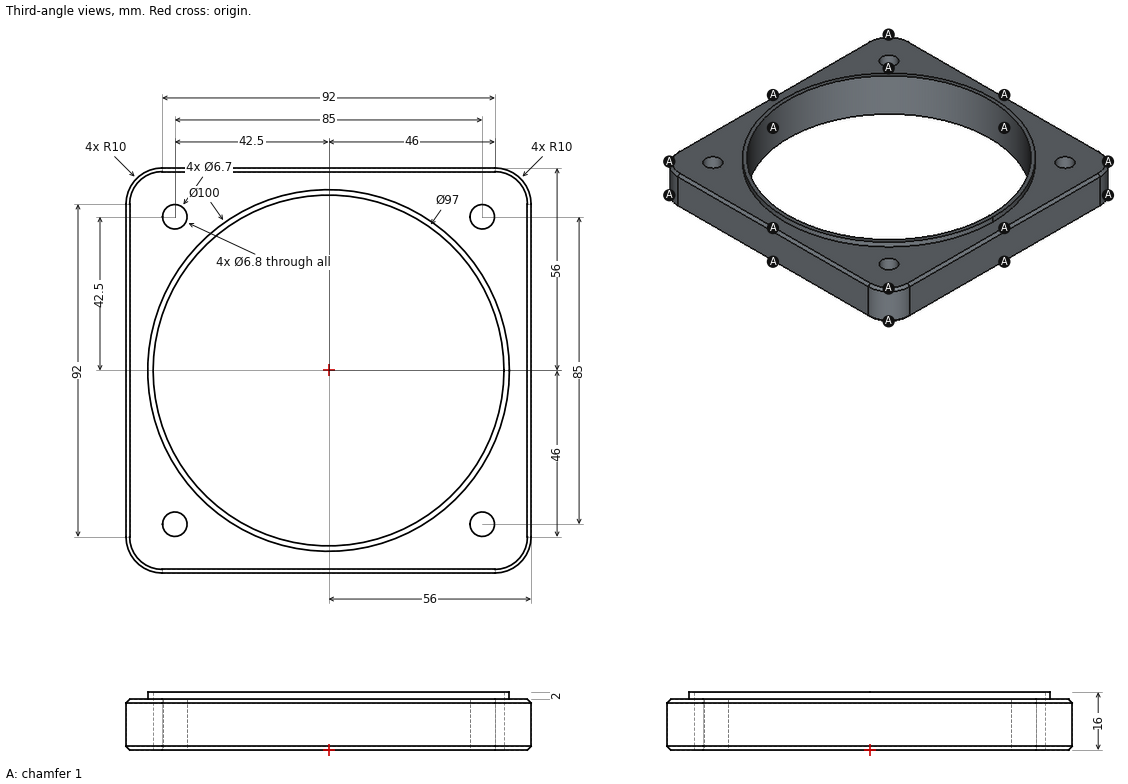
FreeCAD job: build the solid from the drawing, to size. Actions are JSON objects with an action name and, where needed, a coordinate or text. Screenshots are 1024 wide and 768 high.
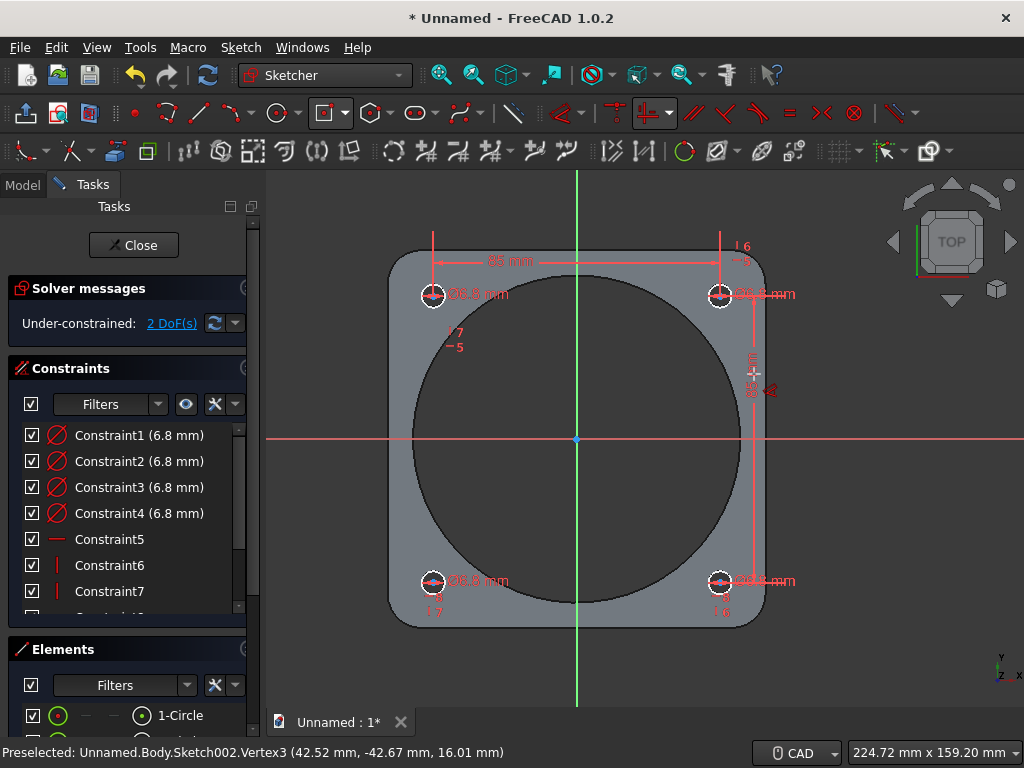
{"action": "left_click", "coordinate": [433, 296]}
{"action": "left_click", "coordinate": [505, 473]}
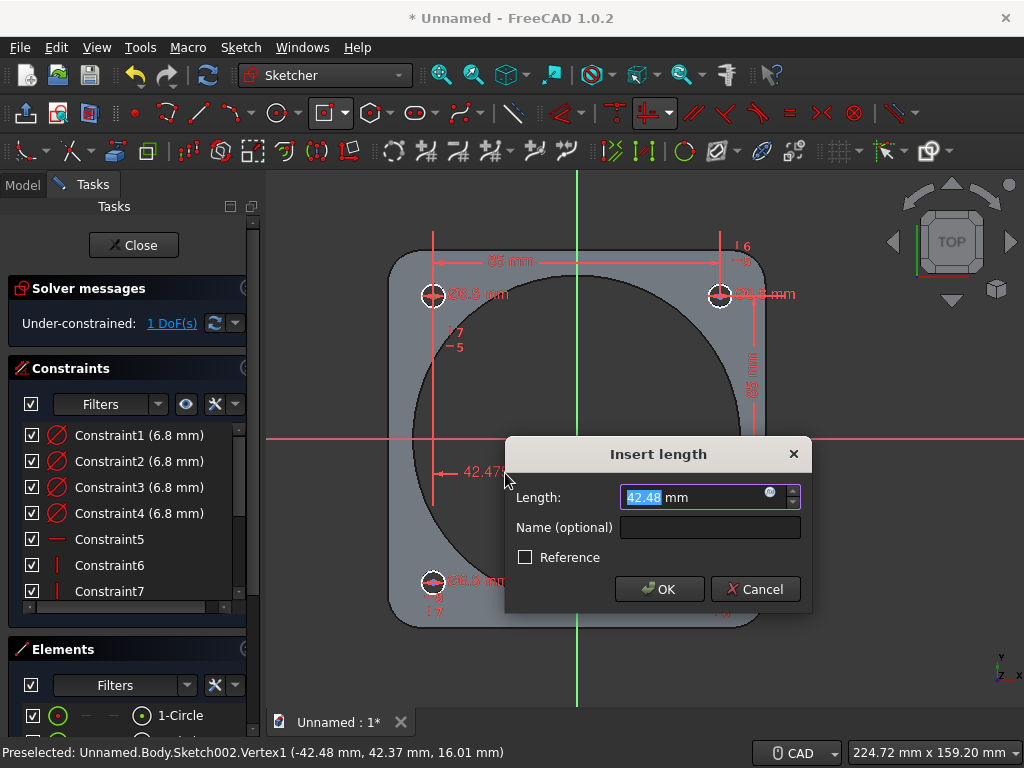
{"action": "type", "text": "42.5"}
{"action": "key", "text": "Return"}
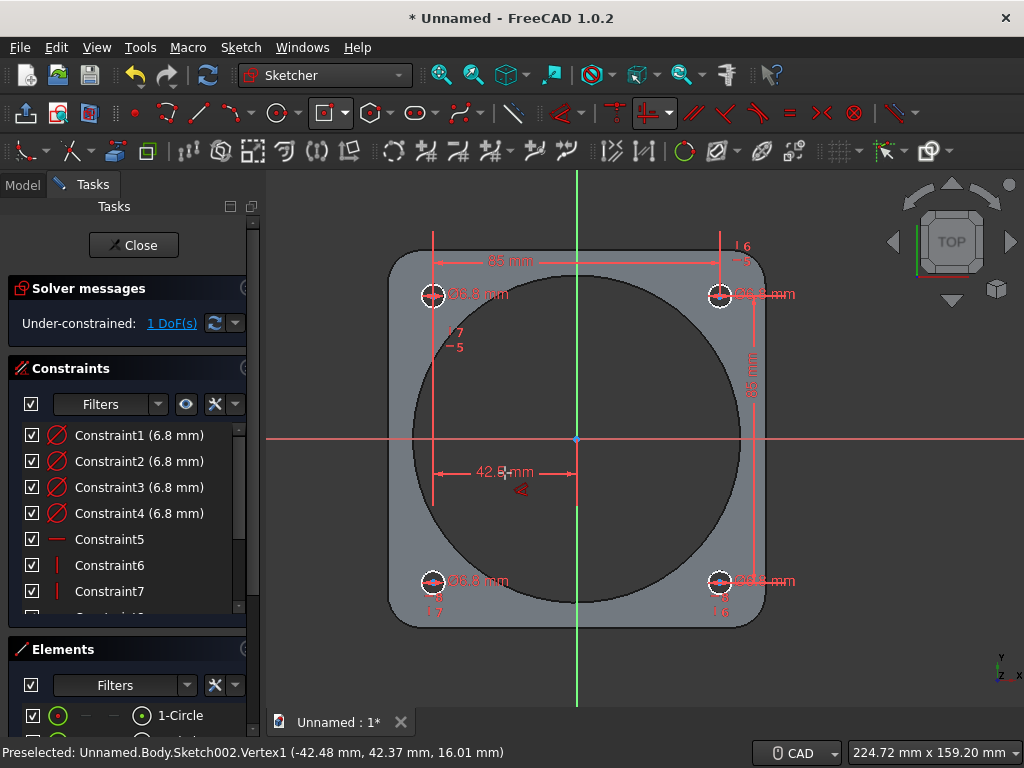
{"action": "left_click", "coordinate": [433, 296]}
{"action": "left_click", "coordinate": [399, 368]}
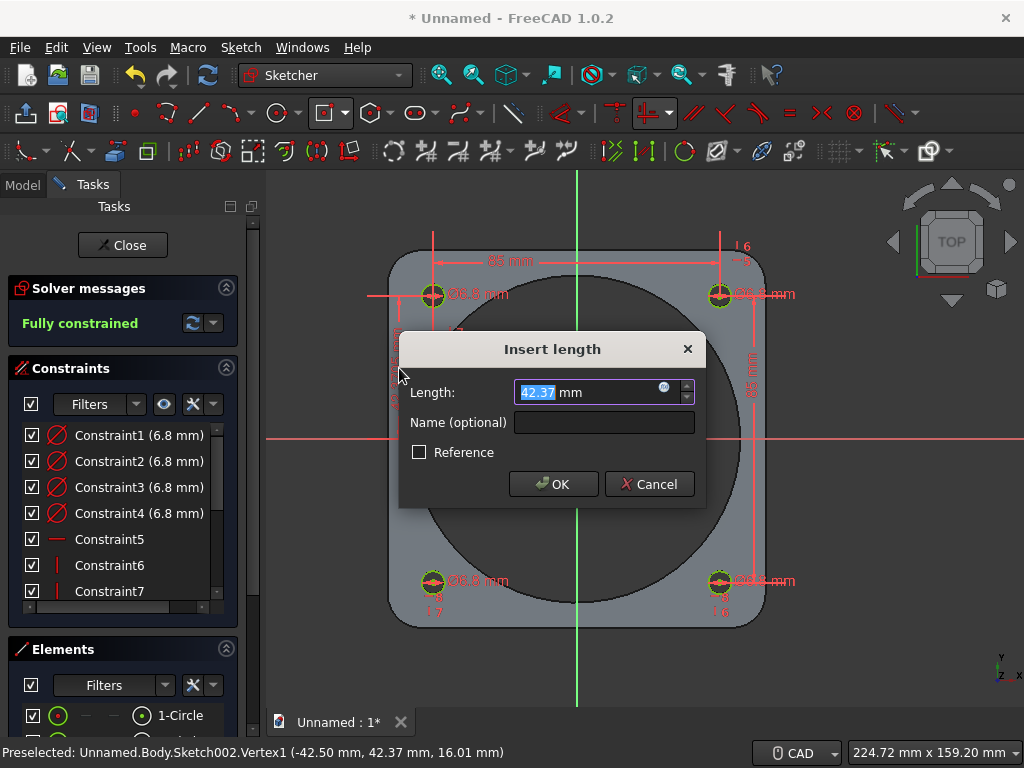
{"action": "type", "text": "42.5"}
{"action": "key", "text": "Return"}
{"action": "key", "text": "Escape"}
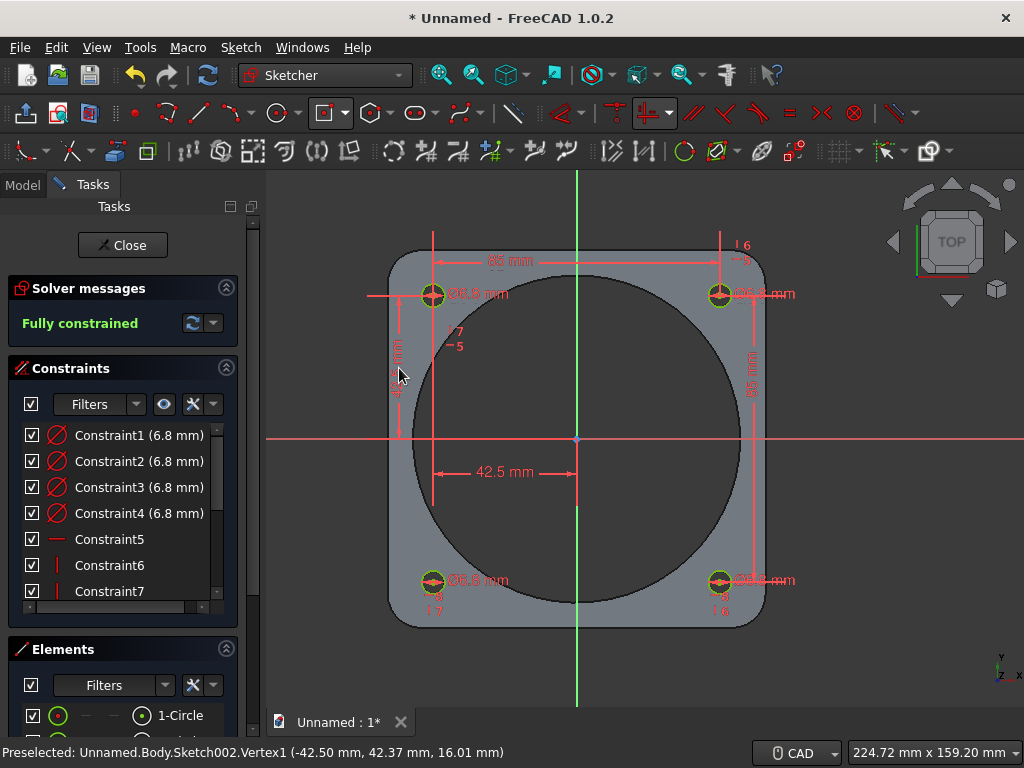
{"action": "left_click", "coordinate": [123, 245]}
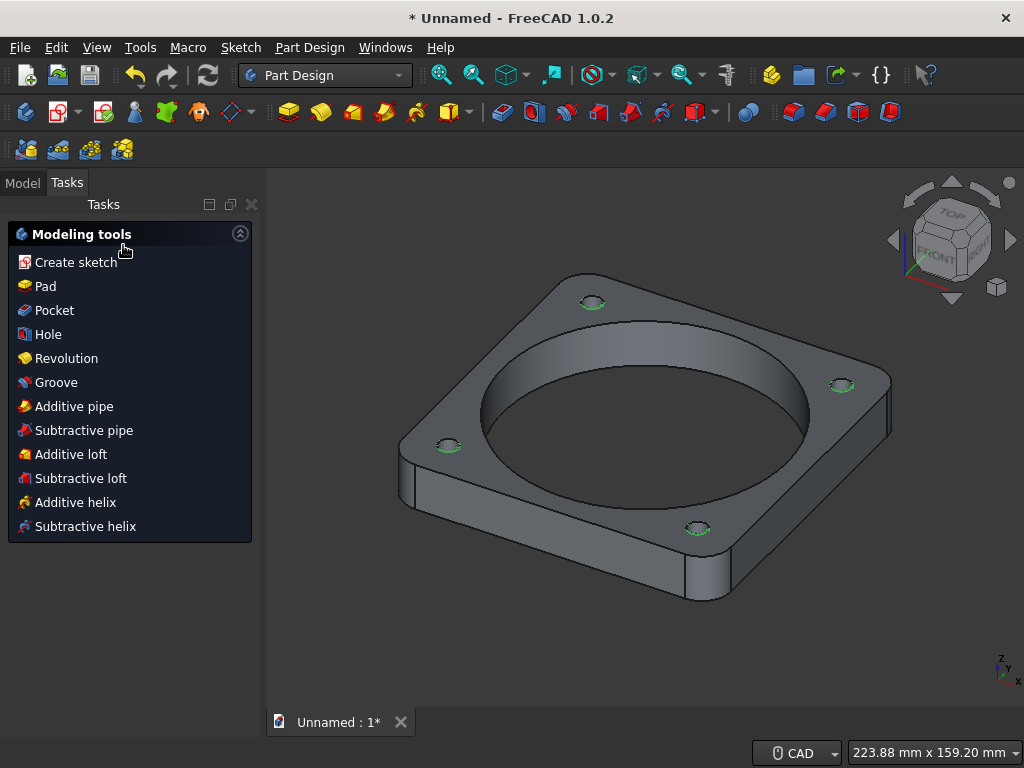
{"action": "left_click", "coordinate": [536, 112]}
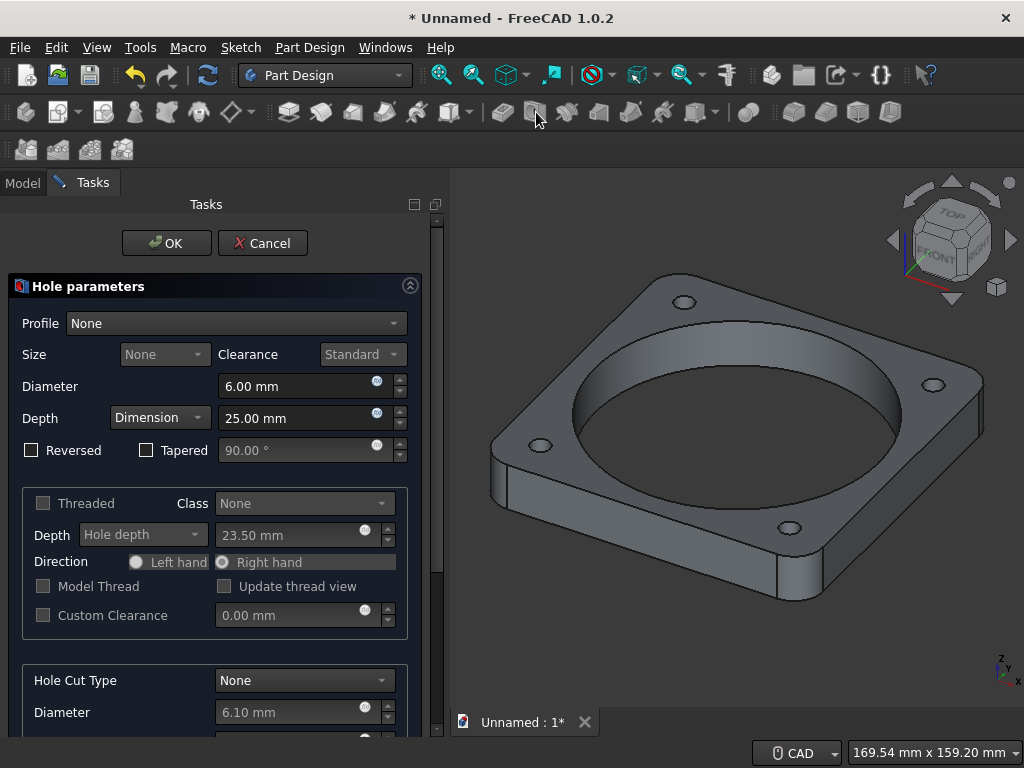
{"action": "triple_click", "coordinate": [305, 386]}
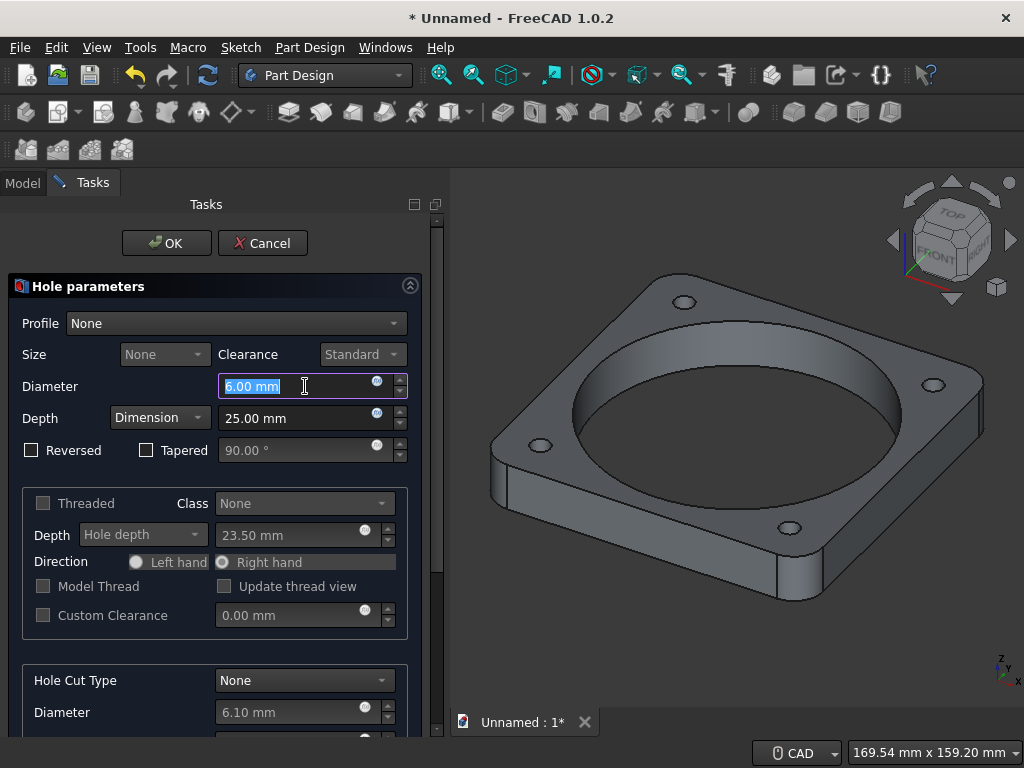
{"action": "type", "text": "6.8"}
{"action": "key", "text": "Tab"}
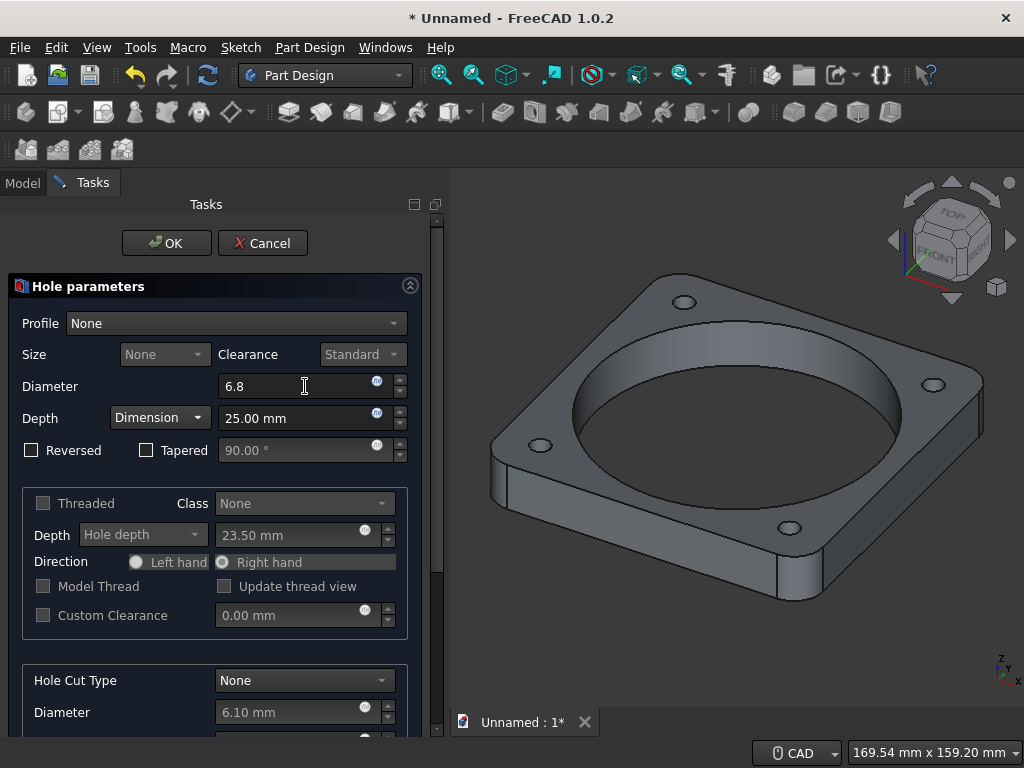
{"action": "left_click", "coordinate": [161, 418]}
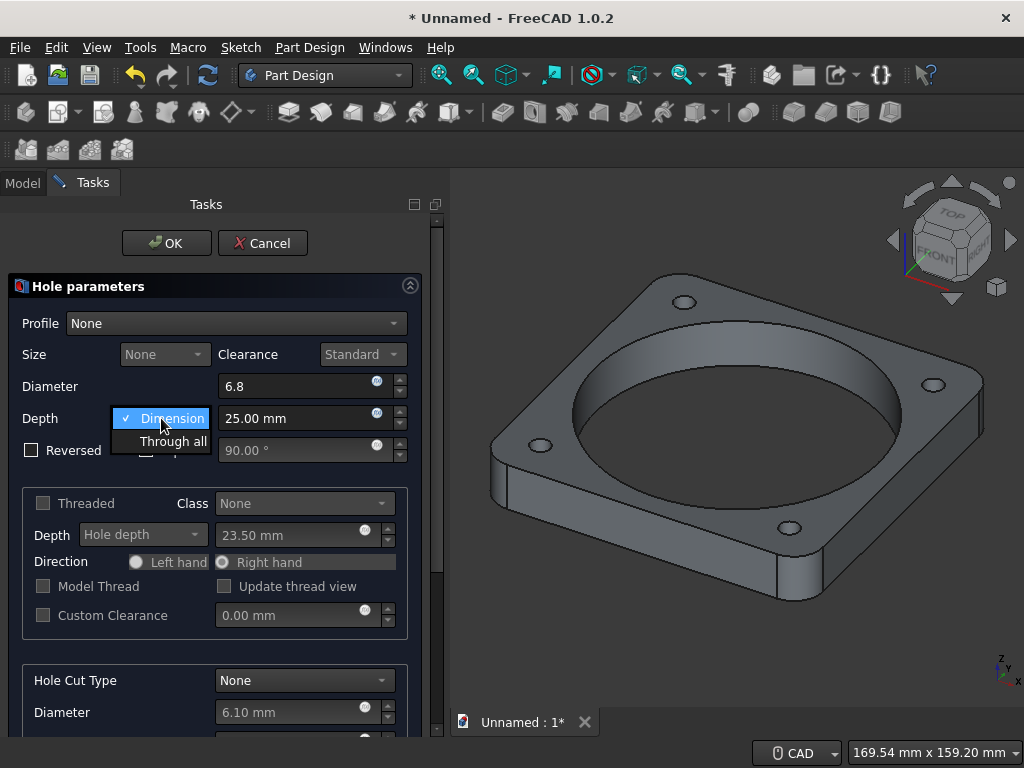
{"action": "left_click", "coordinate": [160, 442]}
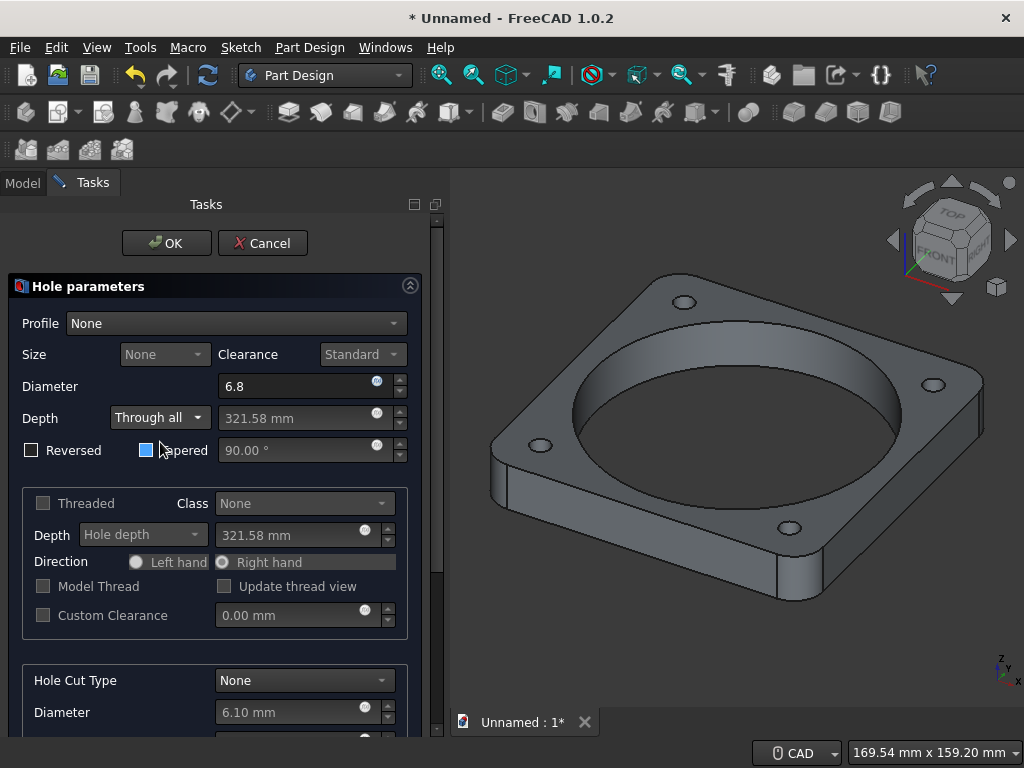
{"action": "left_click", "coordinate": [167, 243]}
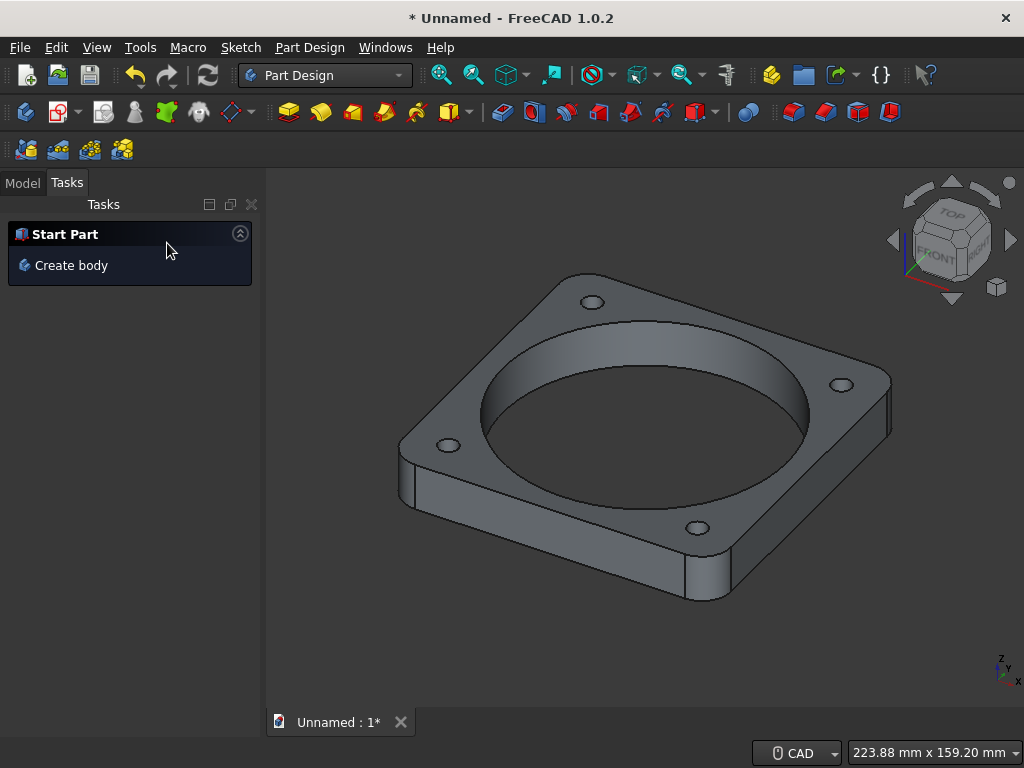
{"action": "left_click", "coordinate": [23, 182]}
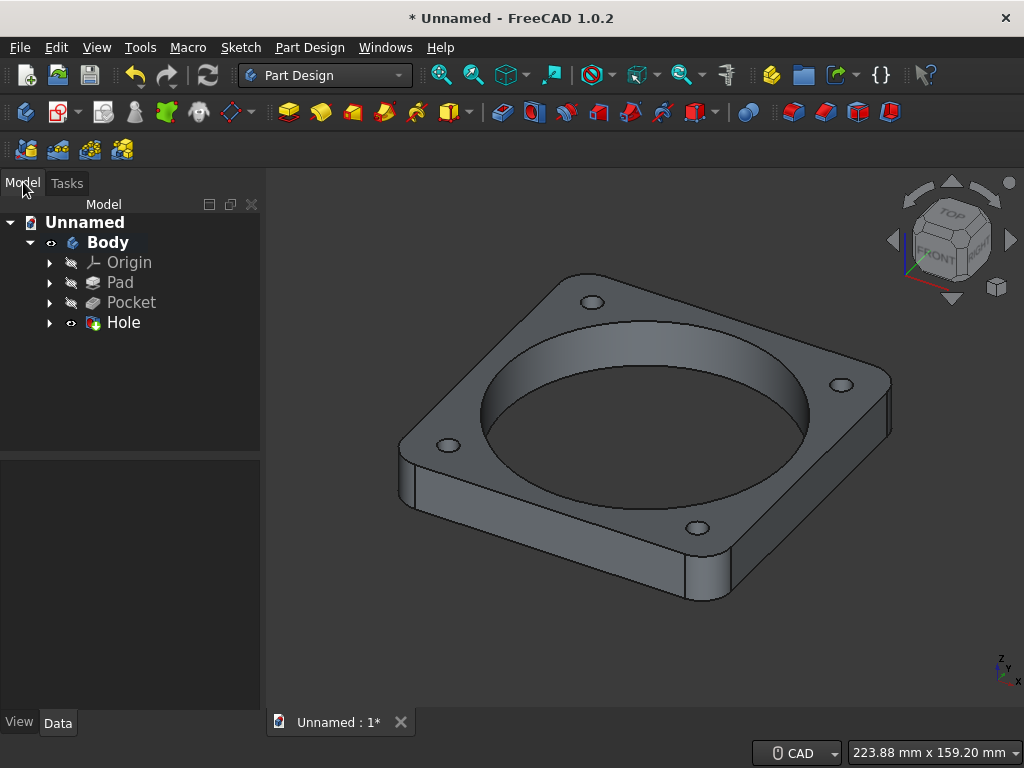
{"action": "left_click", "coordinate": [50, 263]}